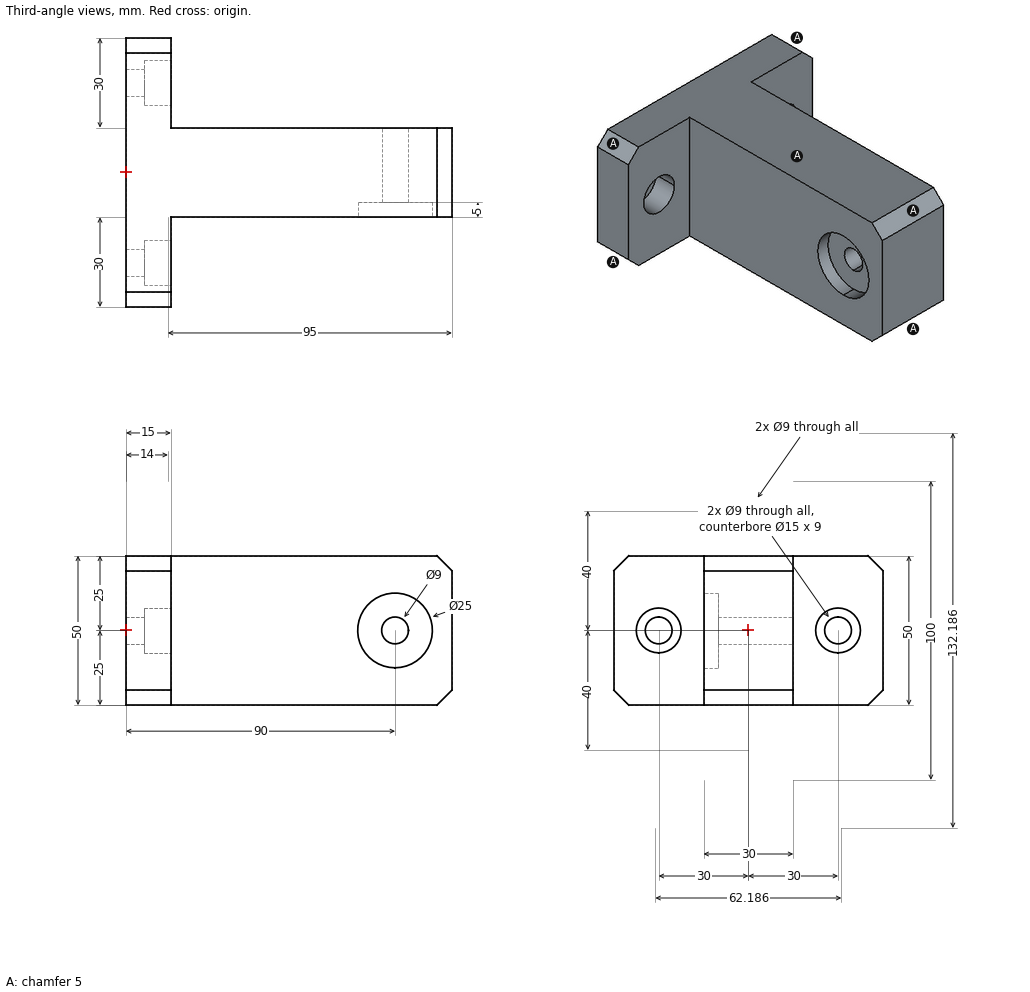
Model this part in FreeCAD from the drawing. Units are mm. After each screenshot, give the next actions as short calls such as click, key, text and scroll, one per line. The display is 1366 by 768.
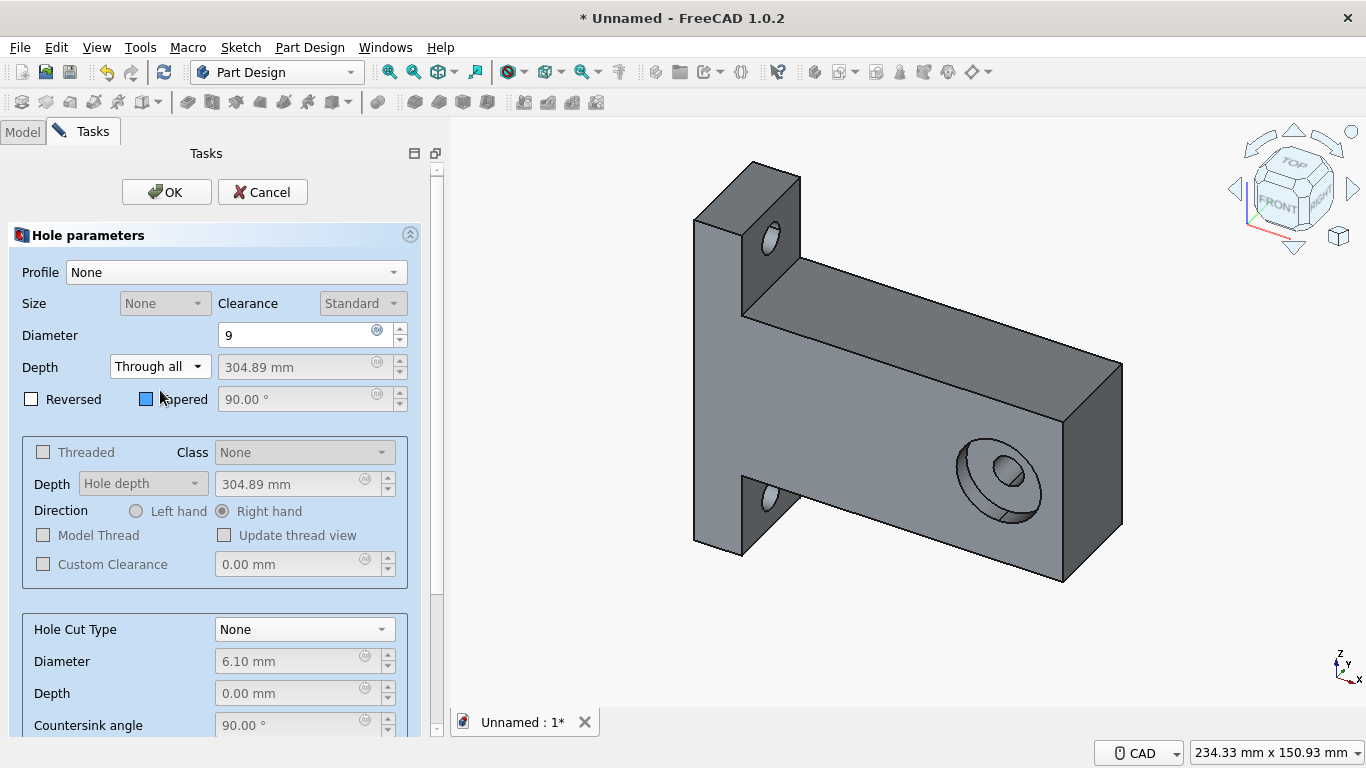
click(167, 192)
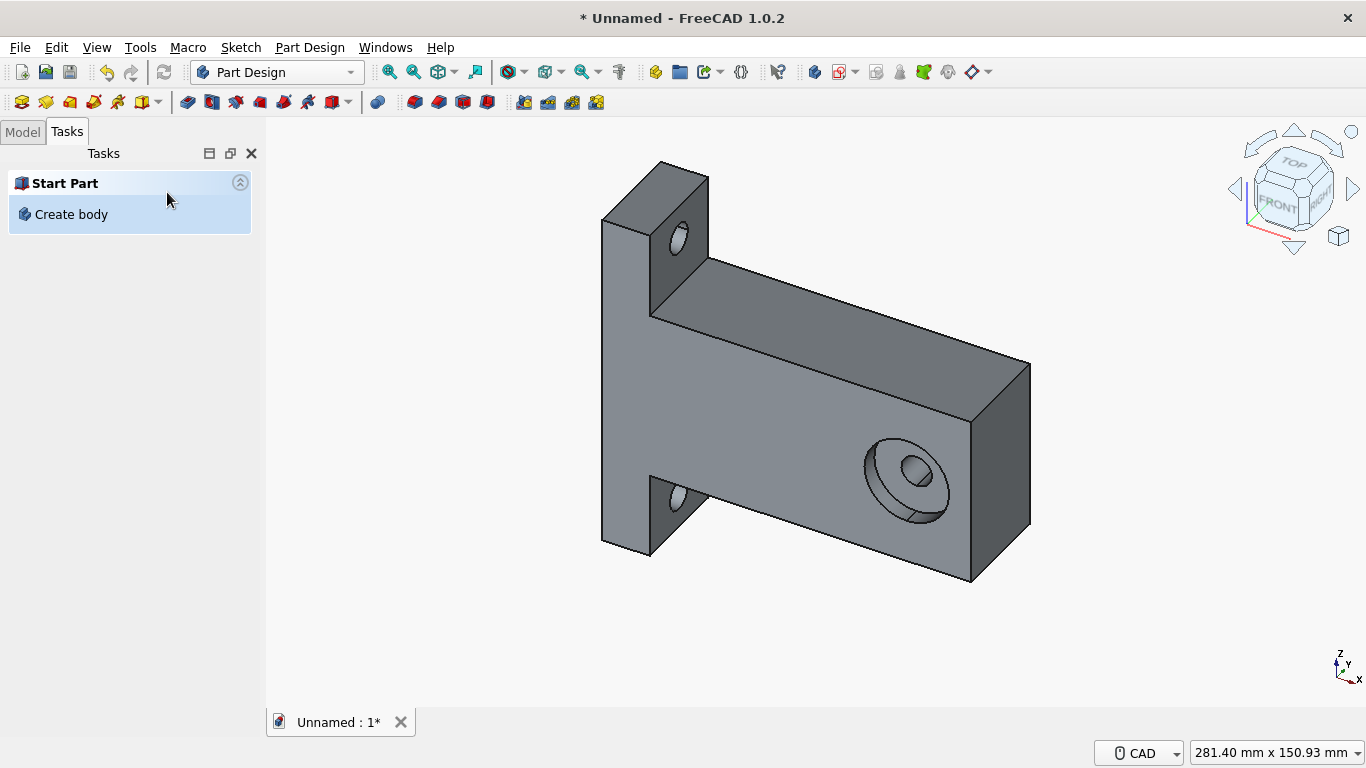
click(1000, 495)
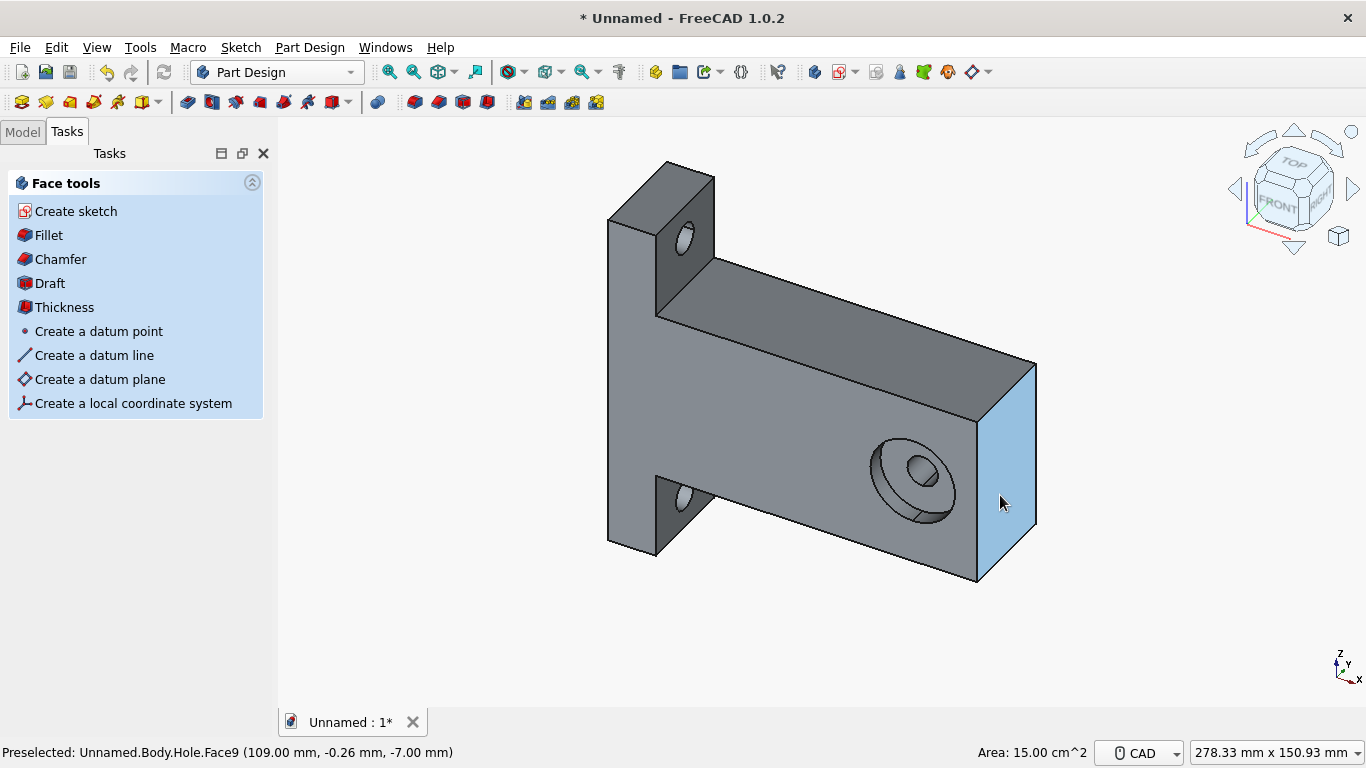
click(840, 72)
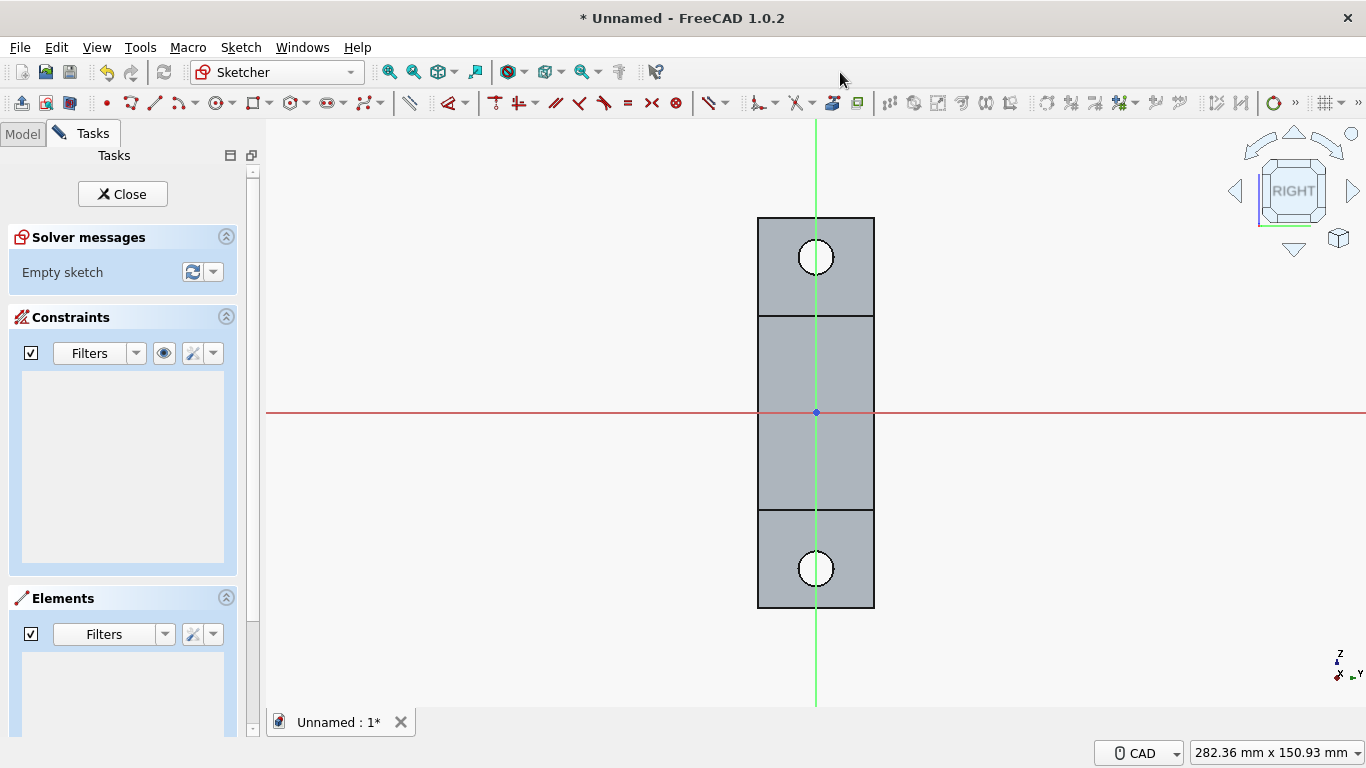
scroll(608, 413, down, 2)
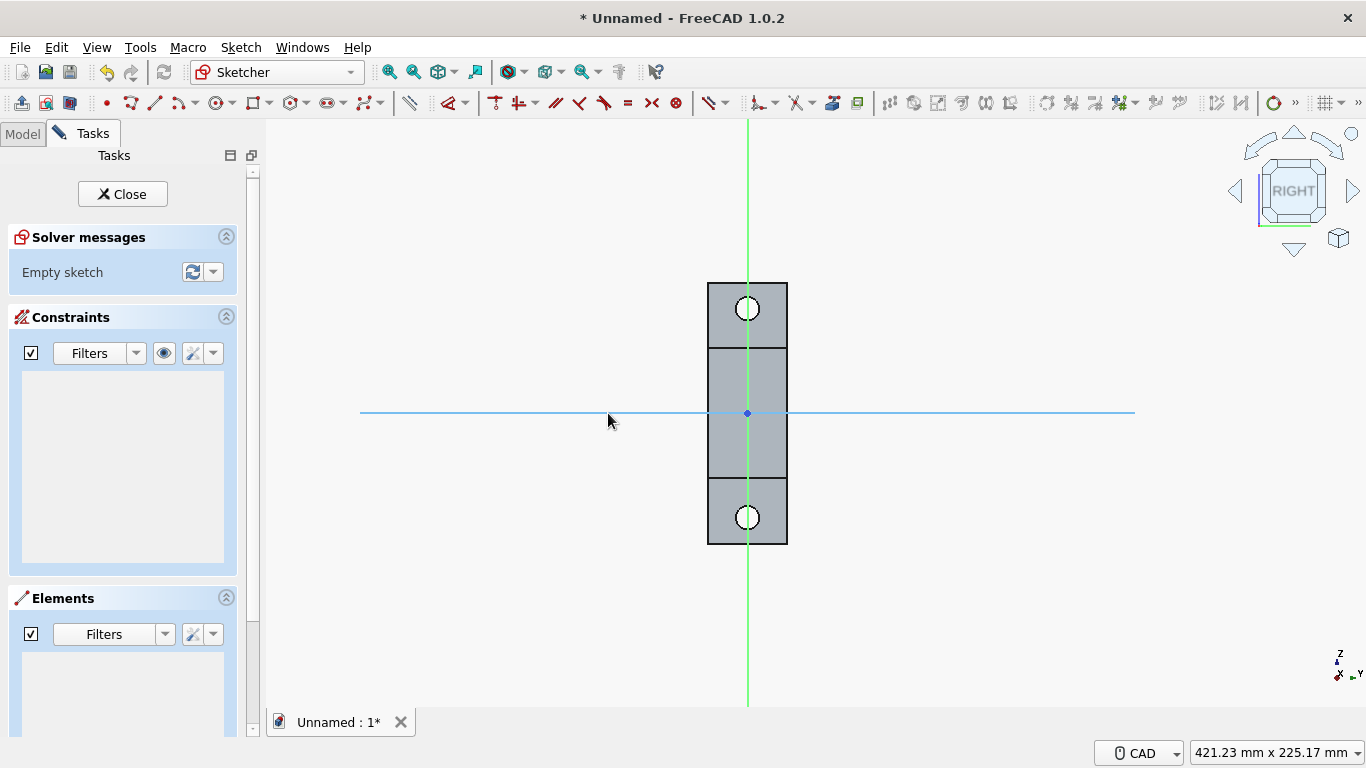
click(272, 104)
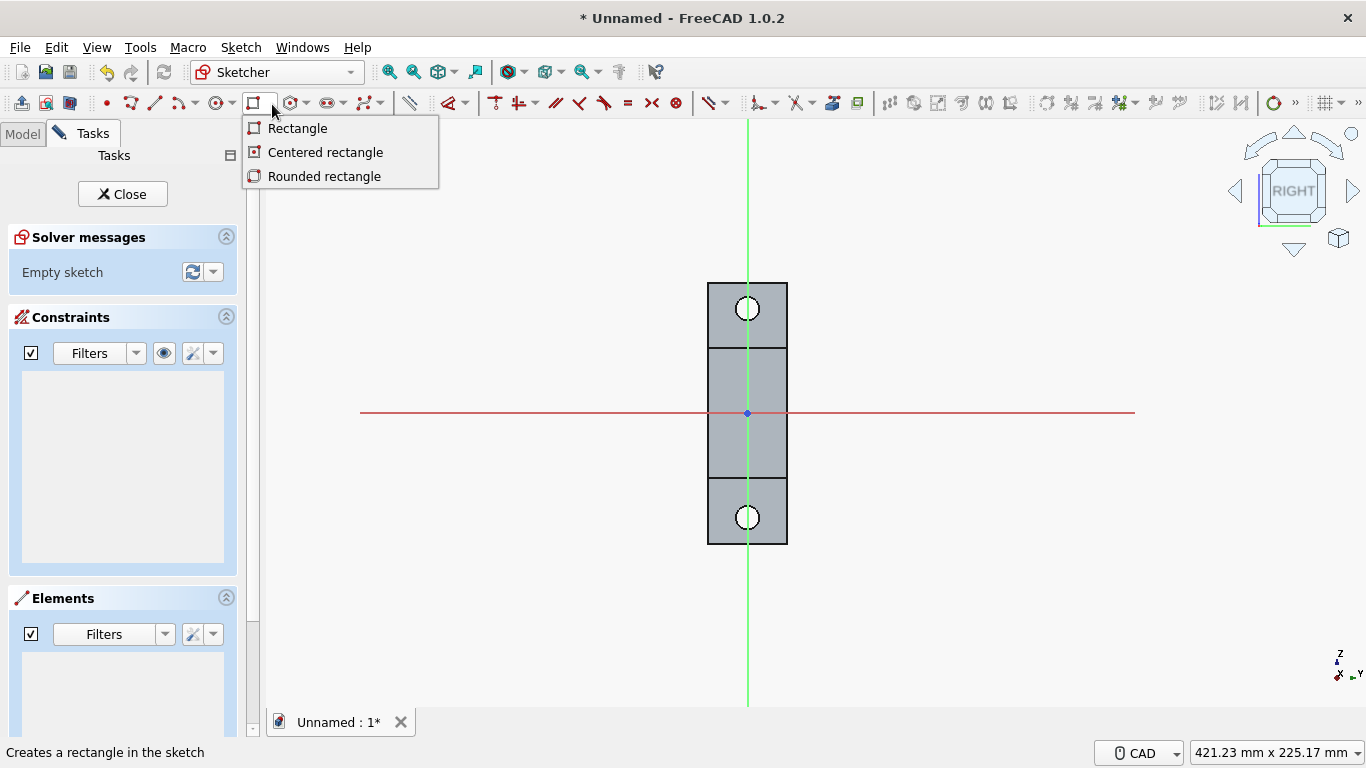
click(340, 152)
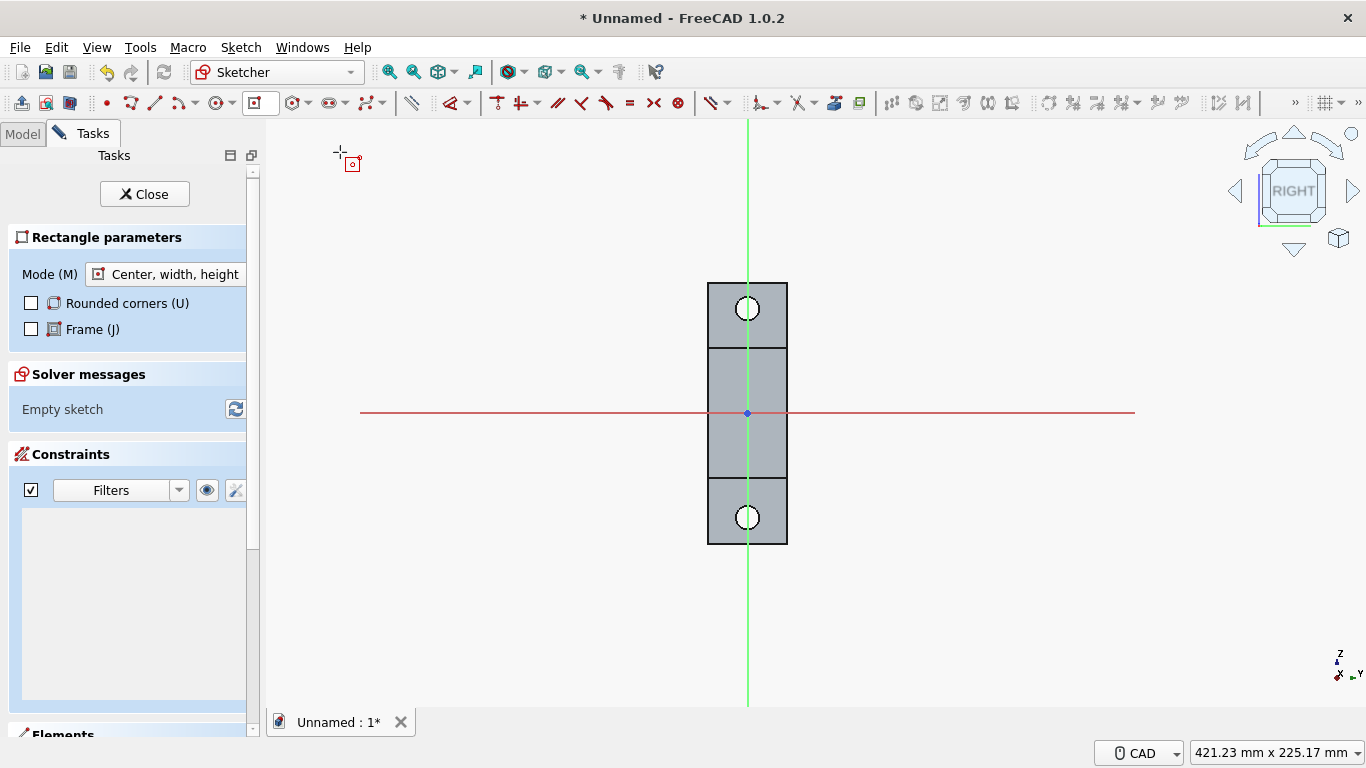
click(748, 413)
move(829, 241)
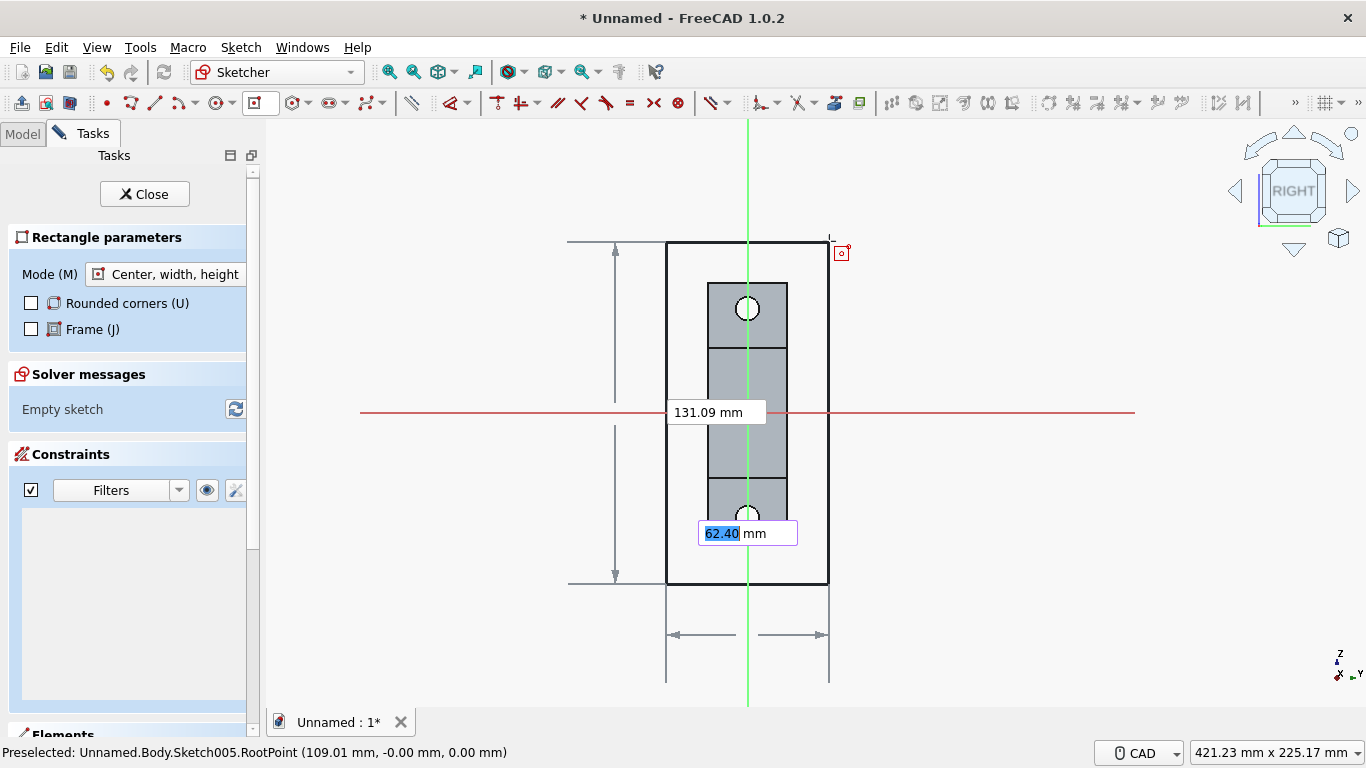
text(62.186)
key(Tab)
text(132.186)
key(Return)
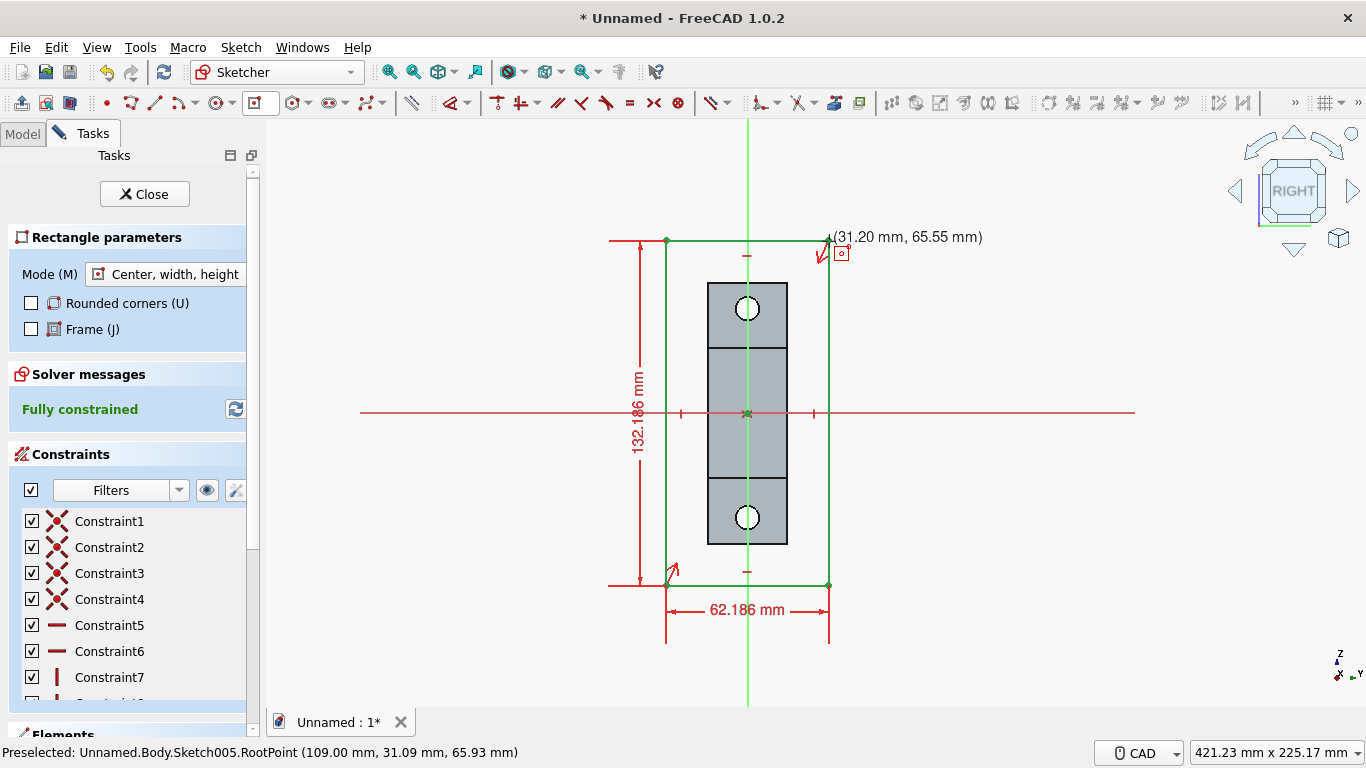
click(748, 413)
move(787, 348)